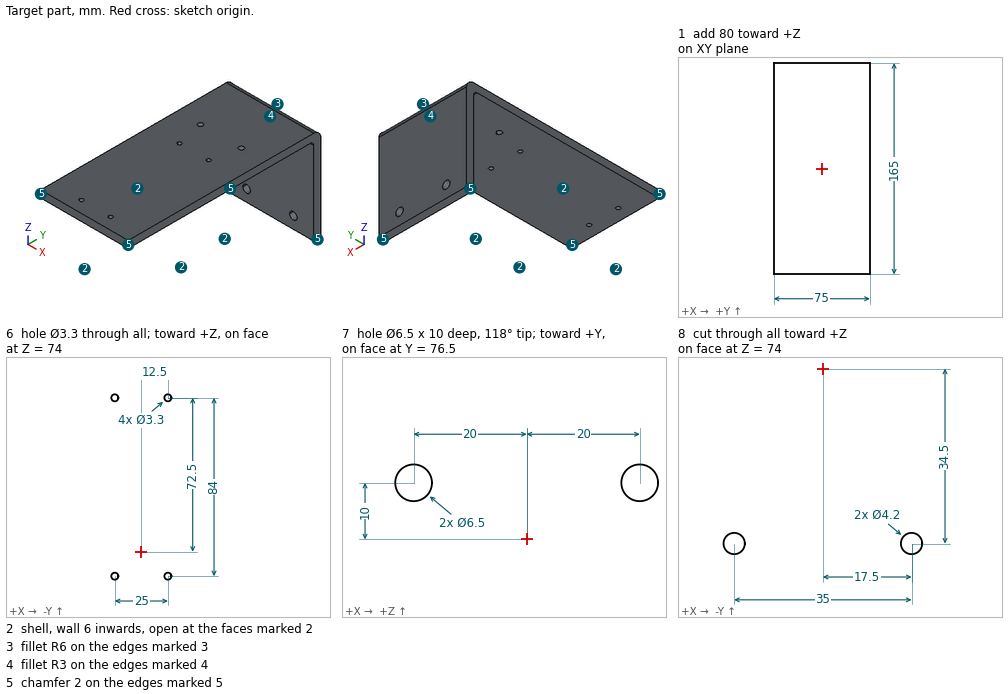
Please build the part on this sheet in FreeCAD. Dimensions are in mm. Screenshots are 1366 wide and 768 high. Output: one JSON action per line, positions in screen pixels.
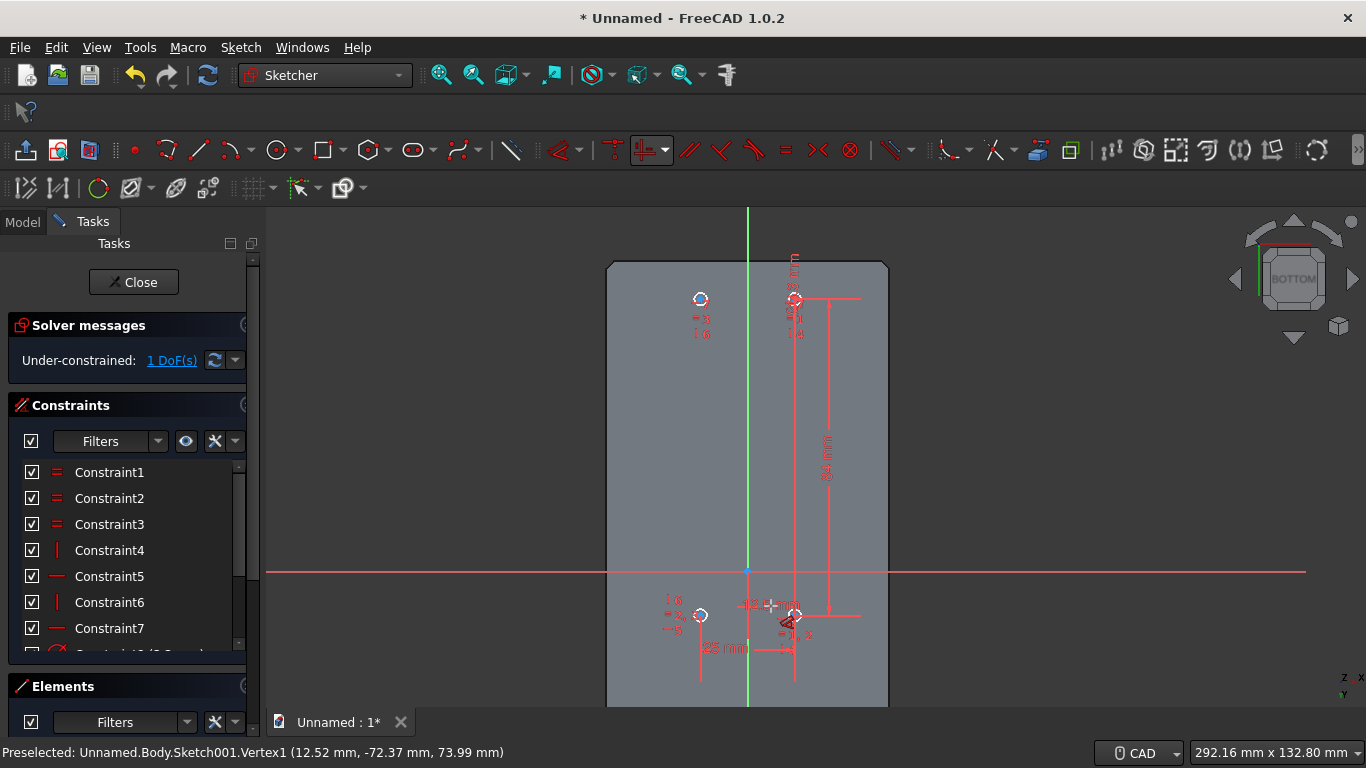
{"action": "left_click", "coordinate": [795, 299]}
{"action": "left_click", "coordinate": [829, 435]}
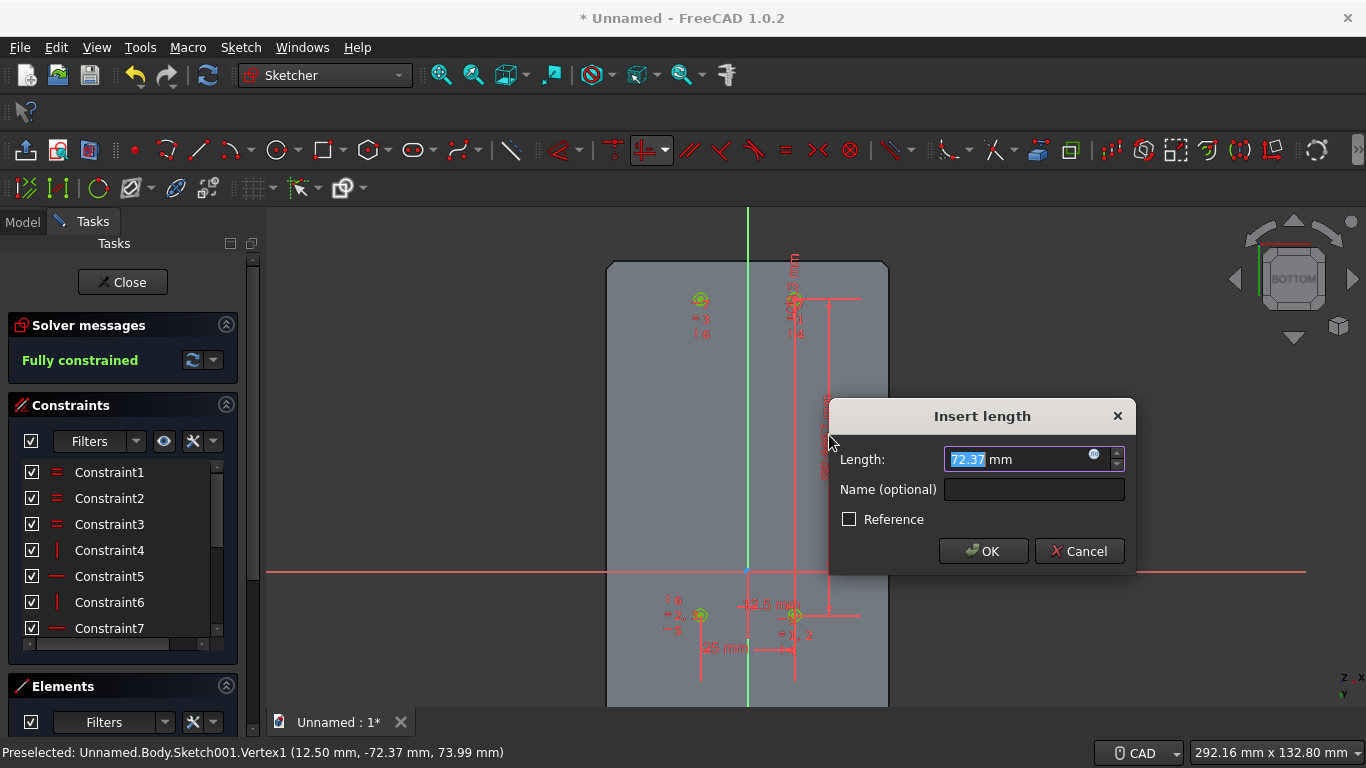
{"action": "type", "text": "72.5"}
{"action": "key", "text": "Return"}
{"action": "key", "text": "Escape"}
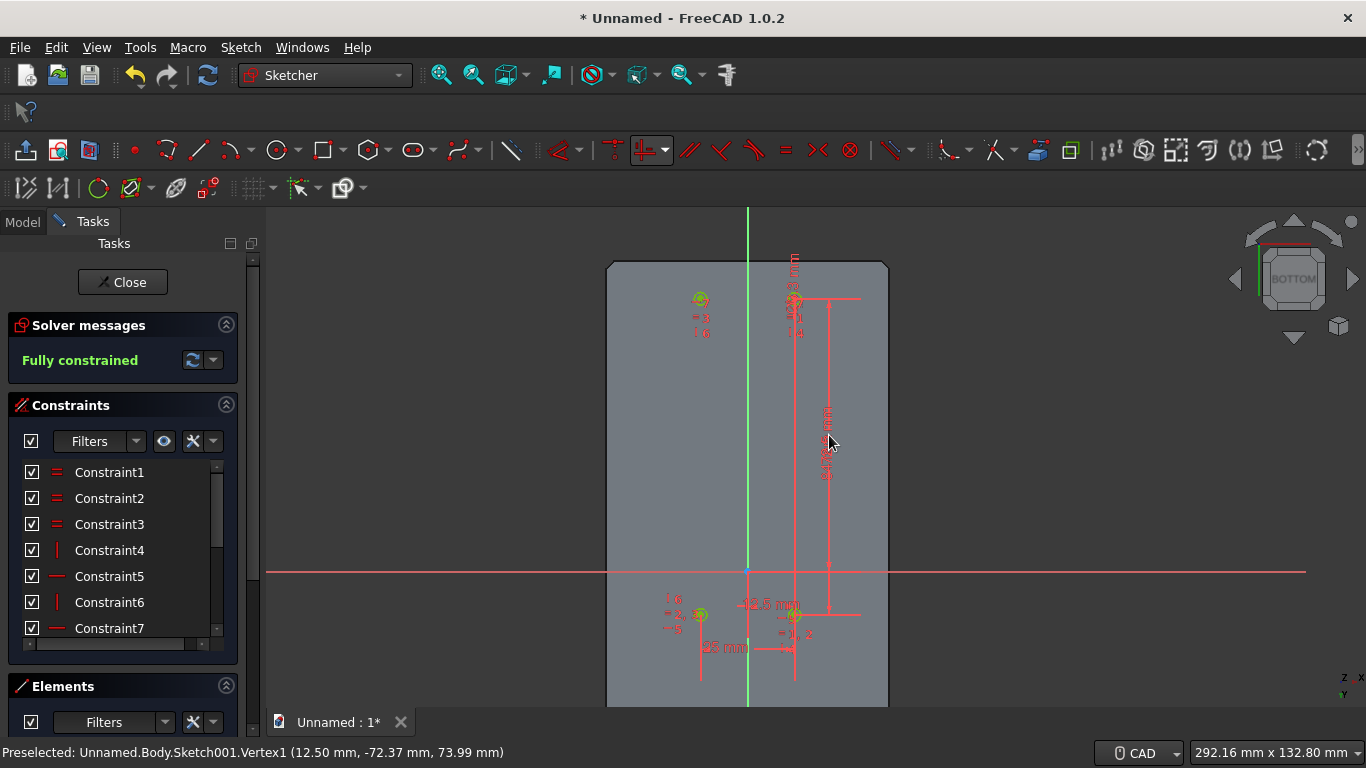
{"action": "left_click", "coordinate": [123, 282]}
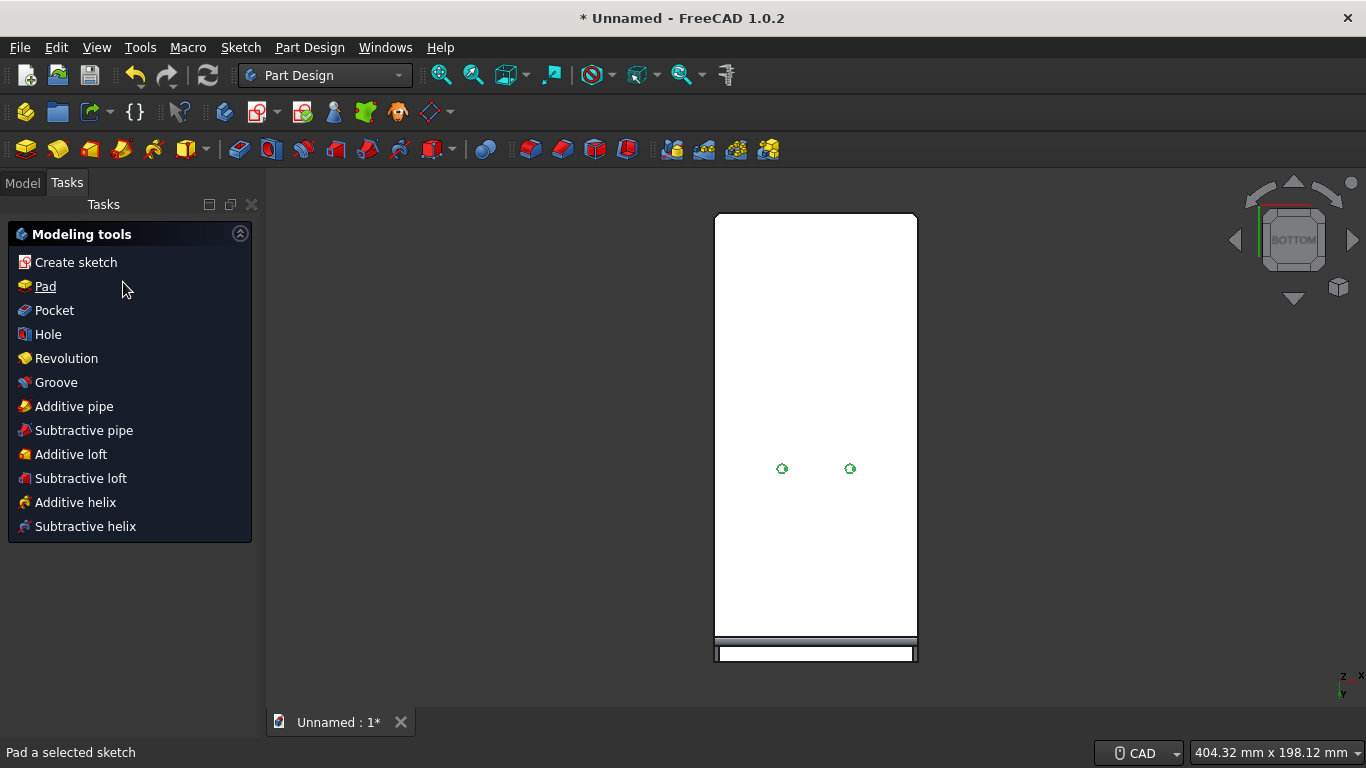
{"action": "left_click", "coordinate": [272, 150]}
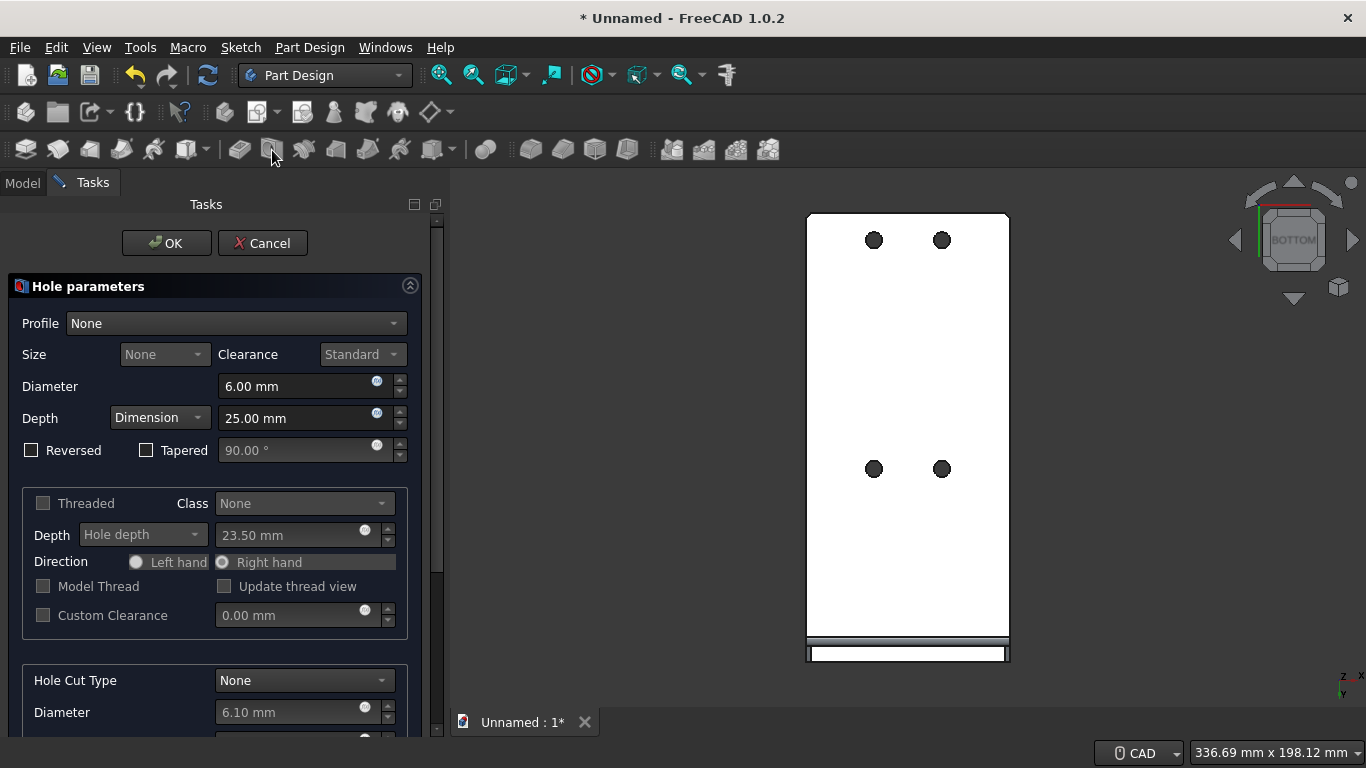
{"action": "triple_click", "coordinate": [305, 386]}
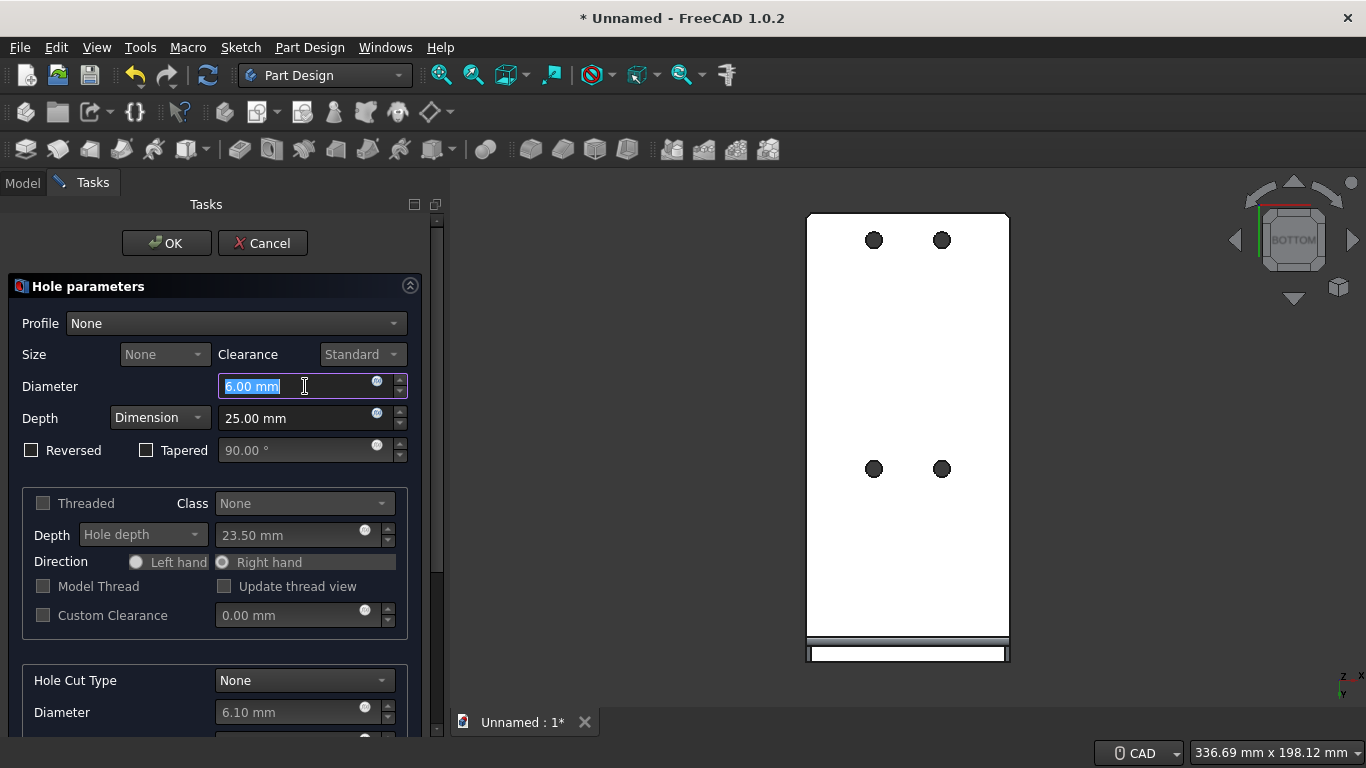
{"action": "type", "text": "3.3"}
{"action": "key", "text": "Tab"}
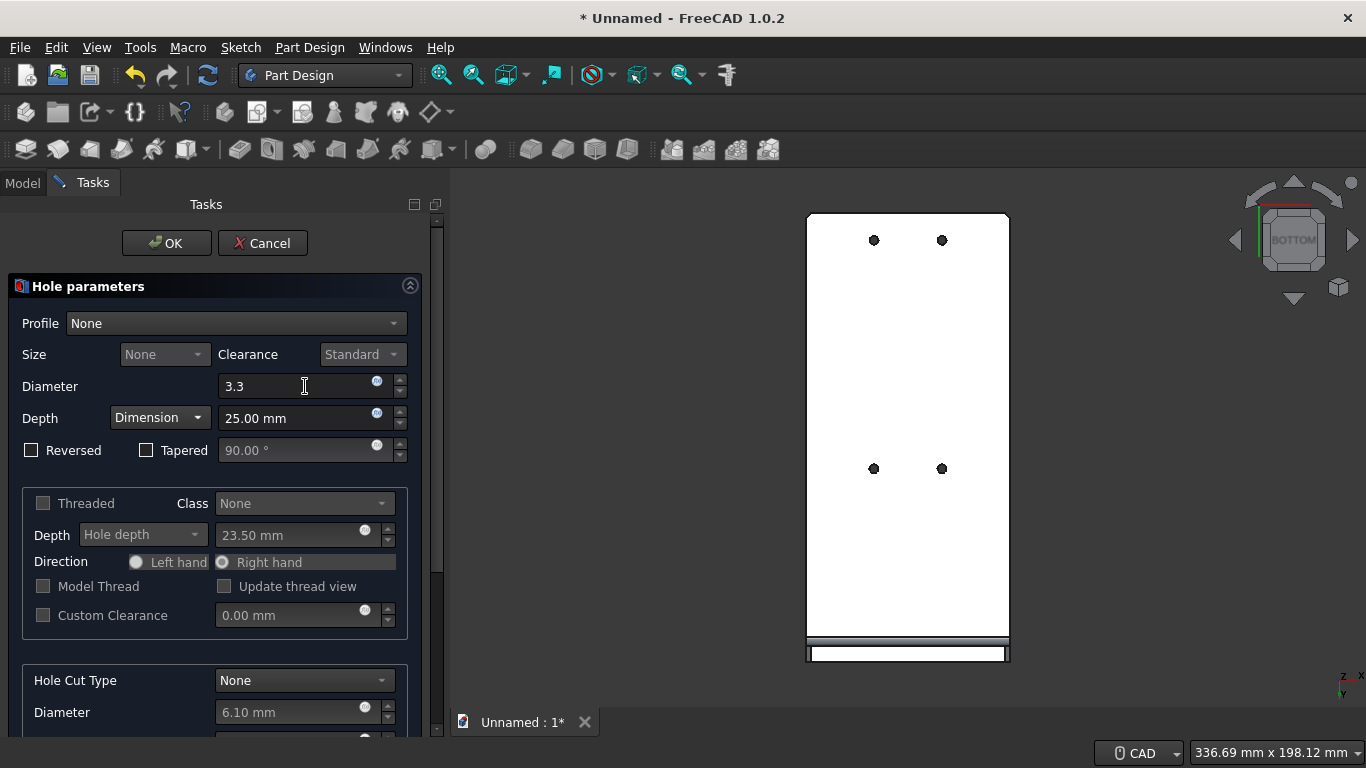
{"action": "left_click", "coordinate": [161, 418]}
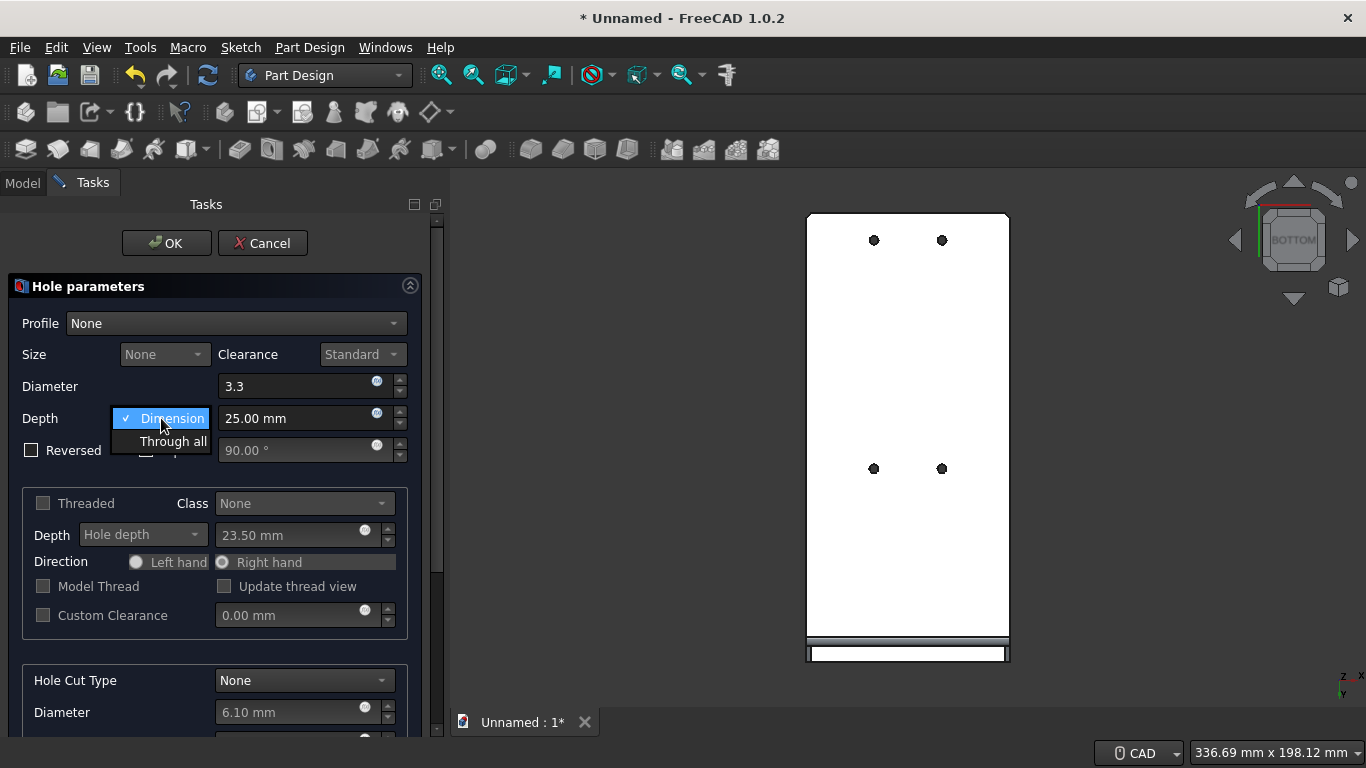
{"action": "left_click", "coordinate": [160, 442]}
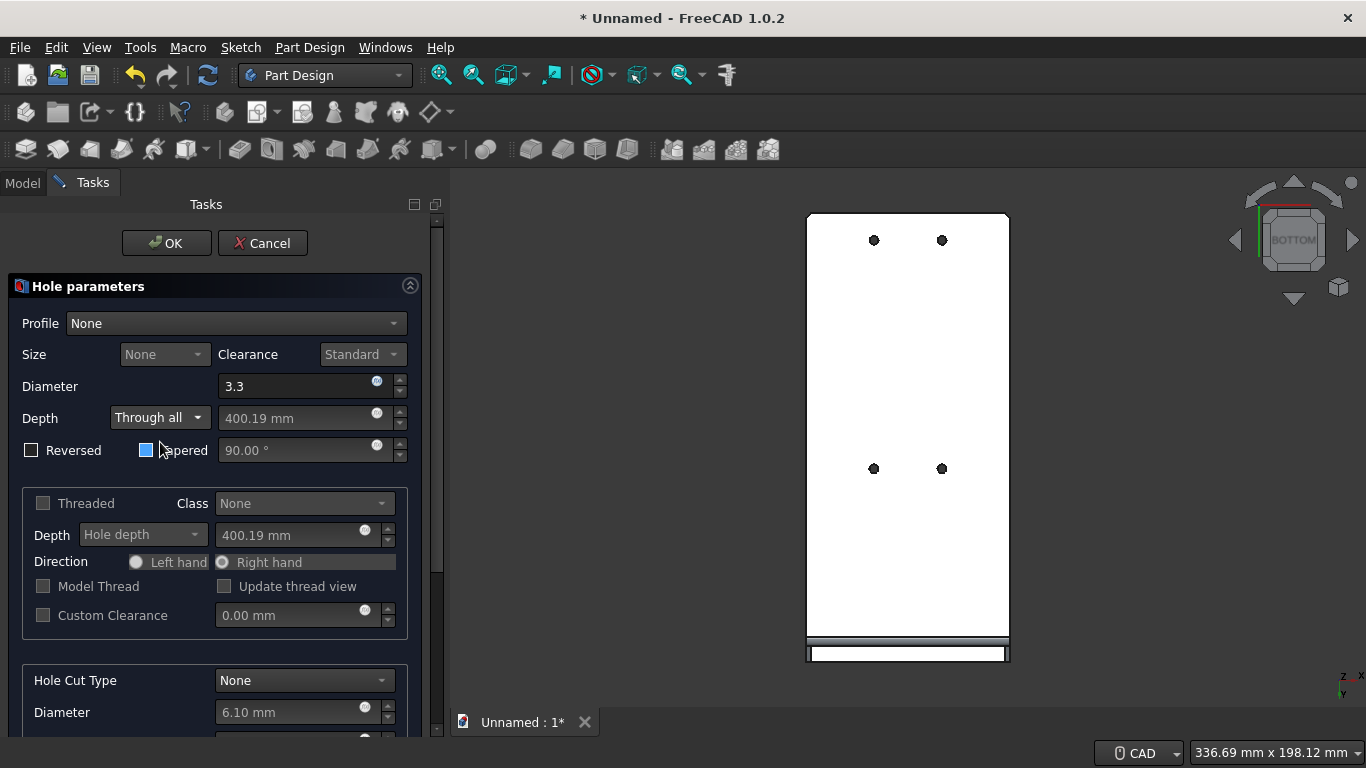
{"action": "left_click", "coordinate": [167, 243]}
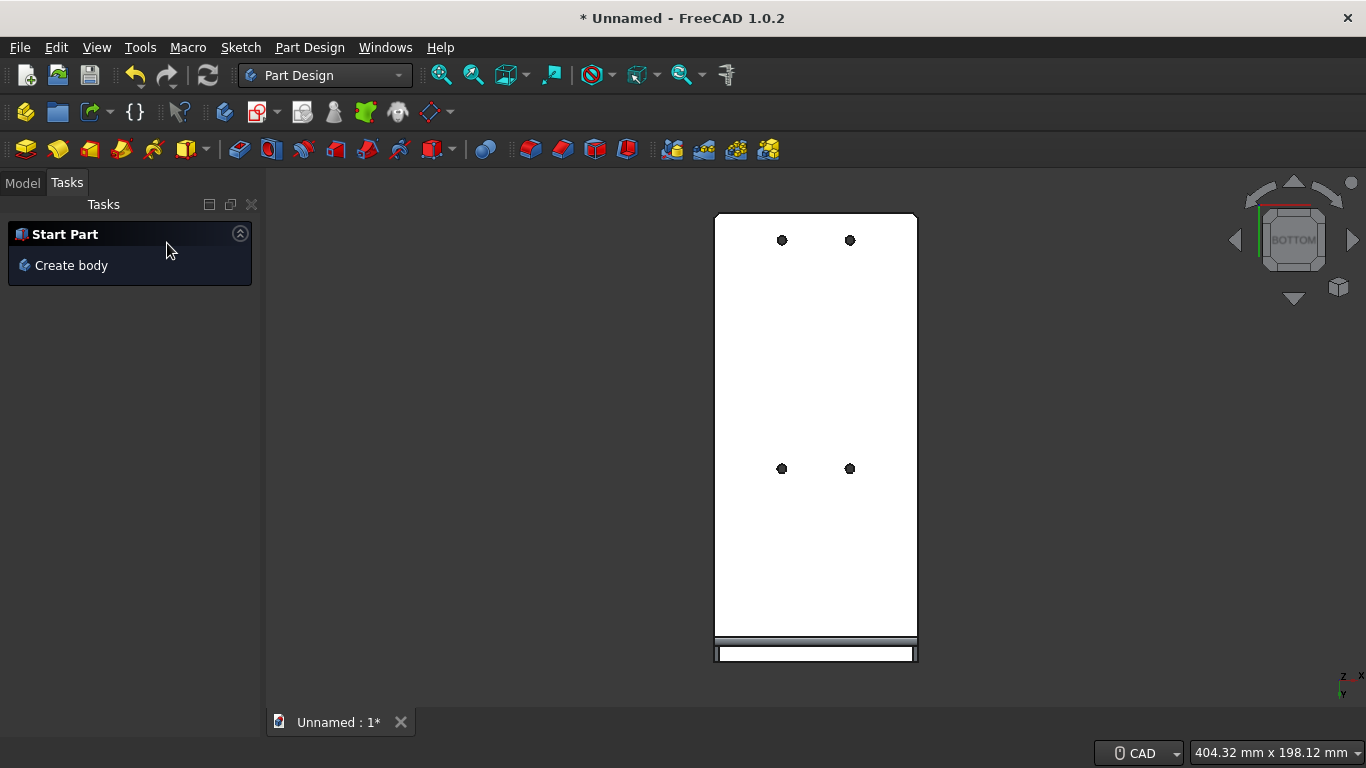
{"action": "key", "text": "0"}